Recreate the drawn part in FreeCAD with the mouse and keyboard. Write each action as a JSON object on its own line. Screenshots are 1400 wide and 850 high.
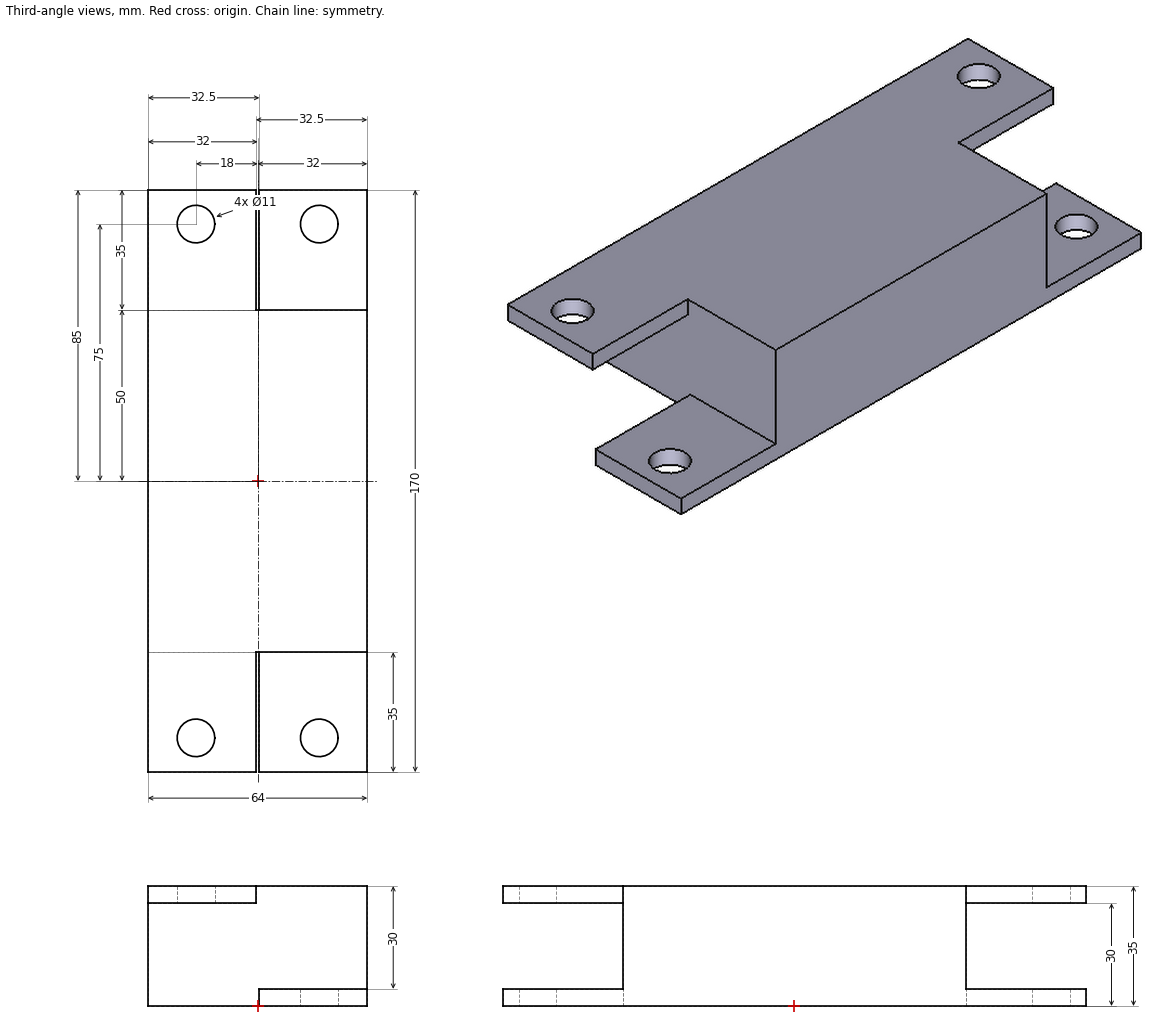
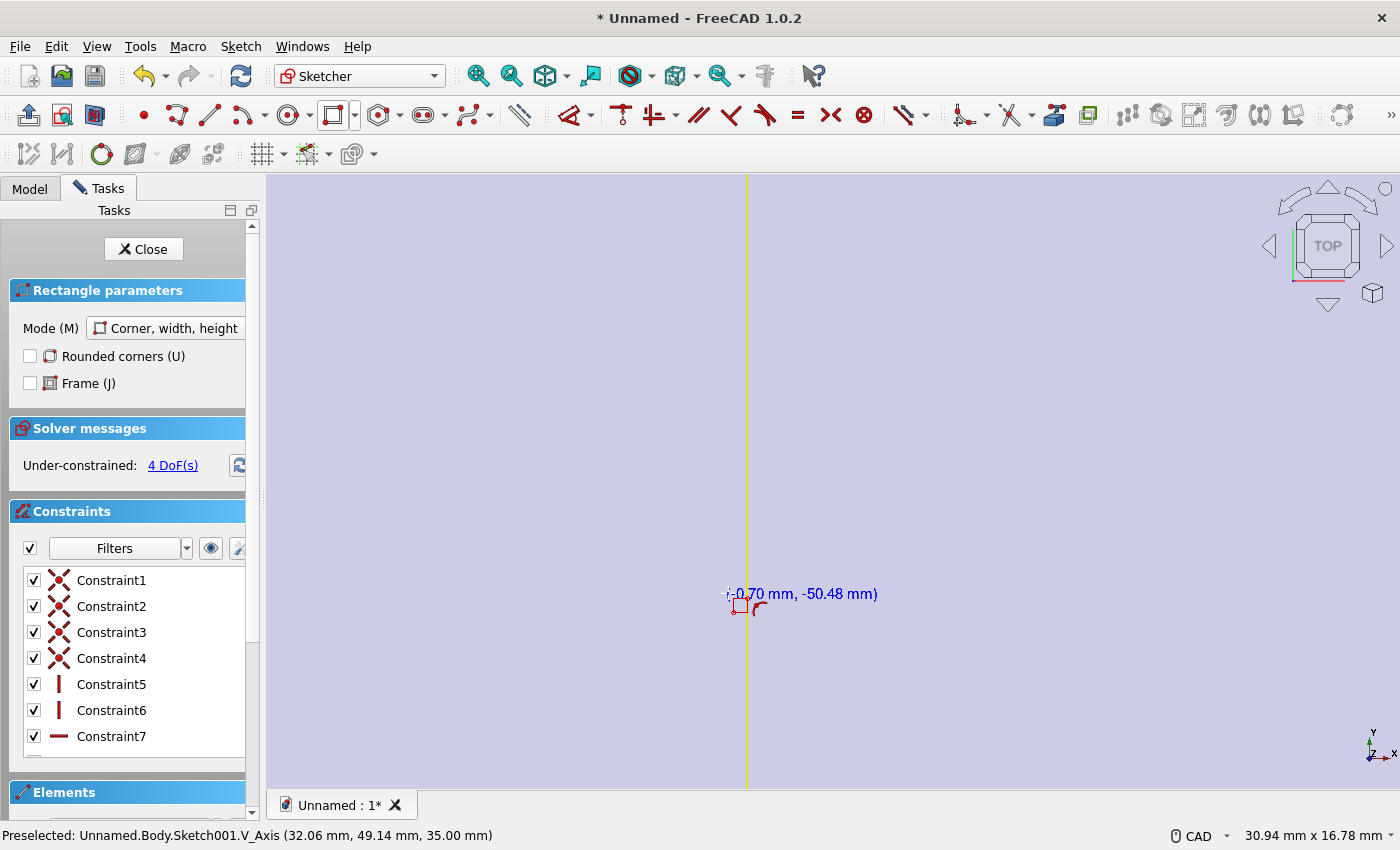
{"action": "left_click", "coordinate": [729, 581]}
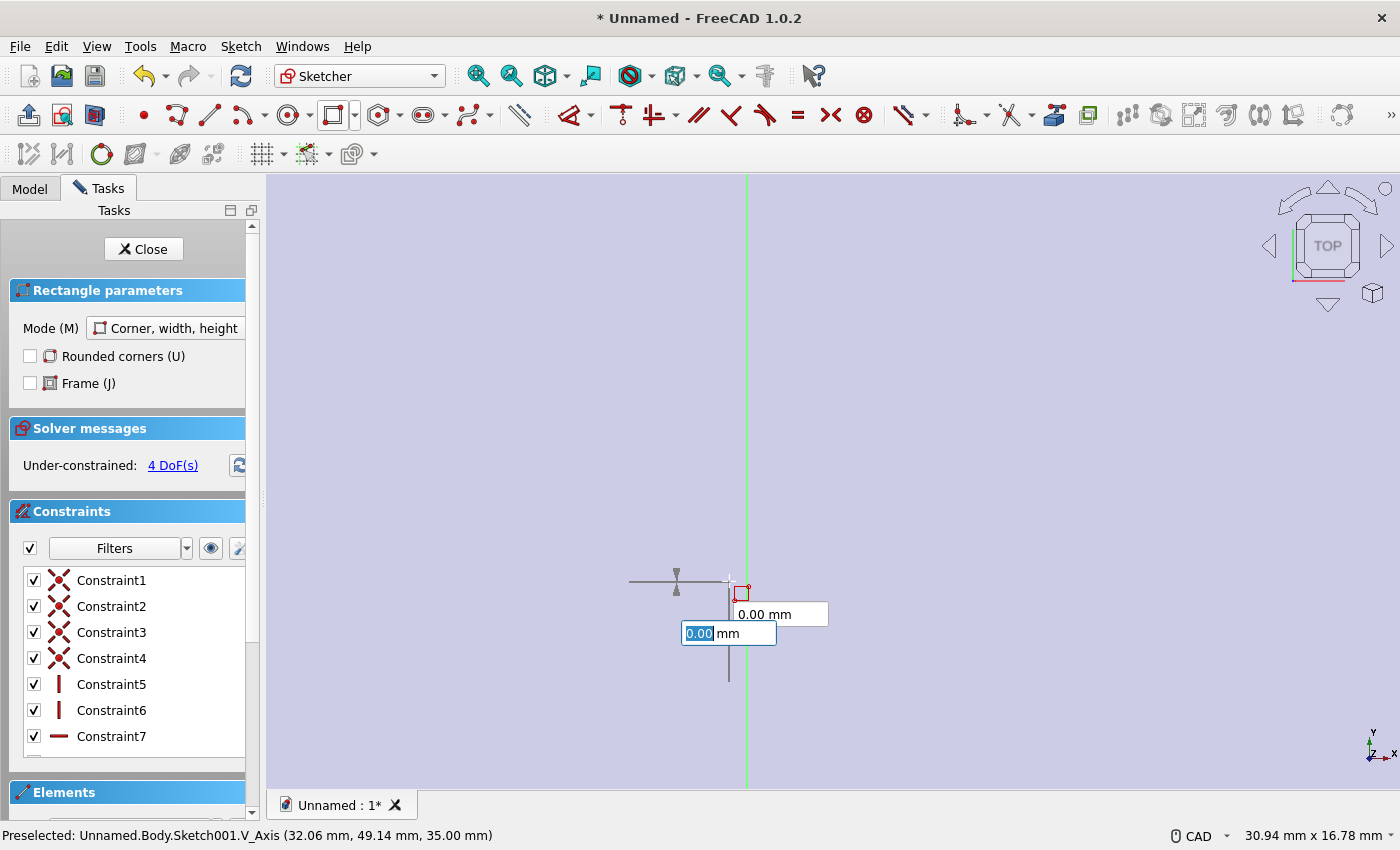
{"action": "scroll", "coordinate": [728, 594], "scroll_direction": "down", "scroll_amount": 14}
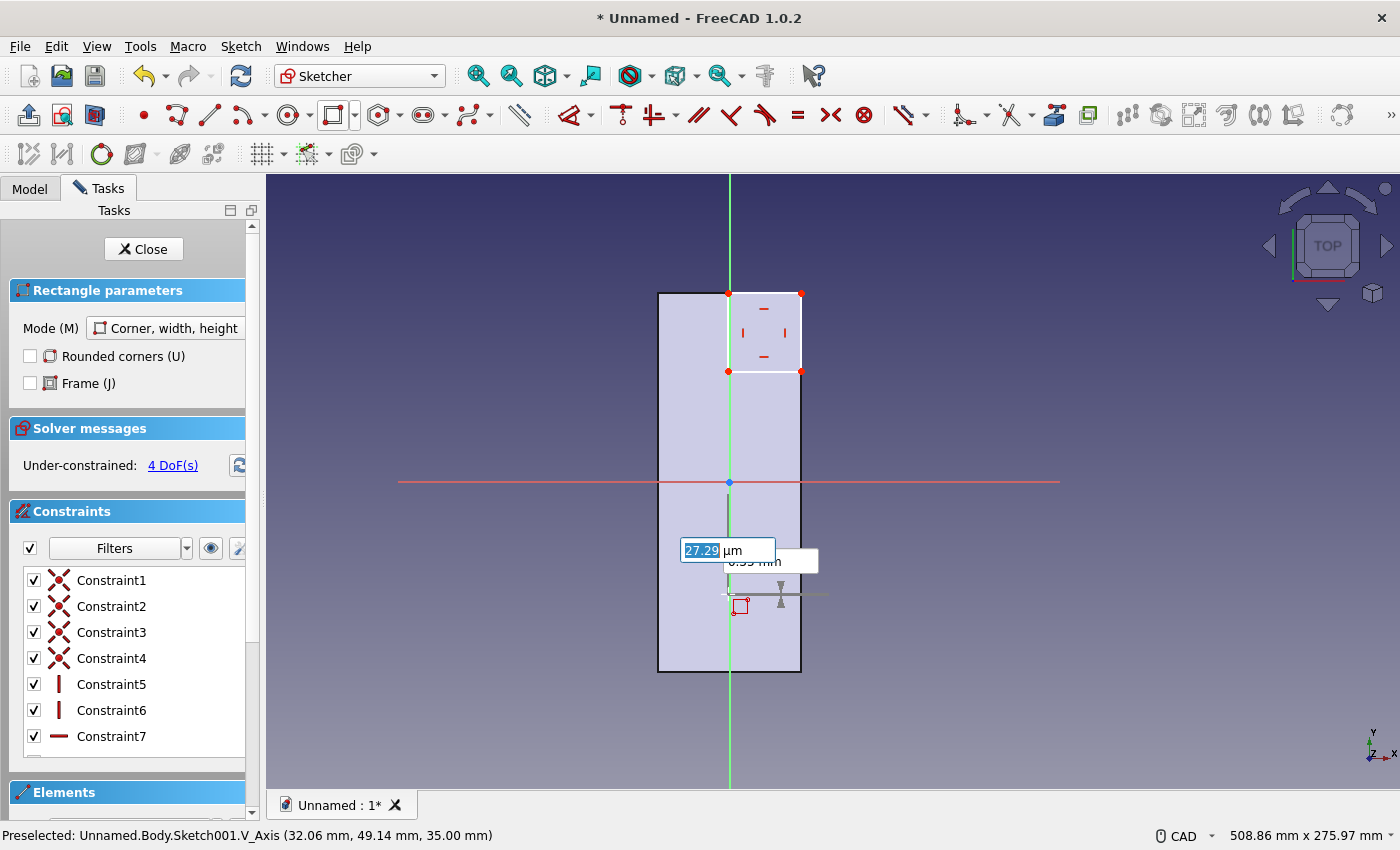
{"action": "left_click", "coordinate": [801, 672]}
{"action": "key", "text": "Escape"}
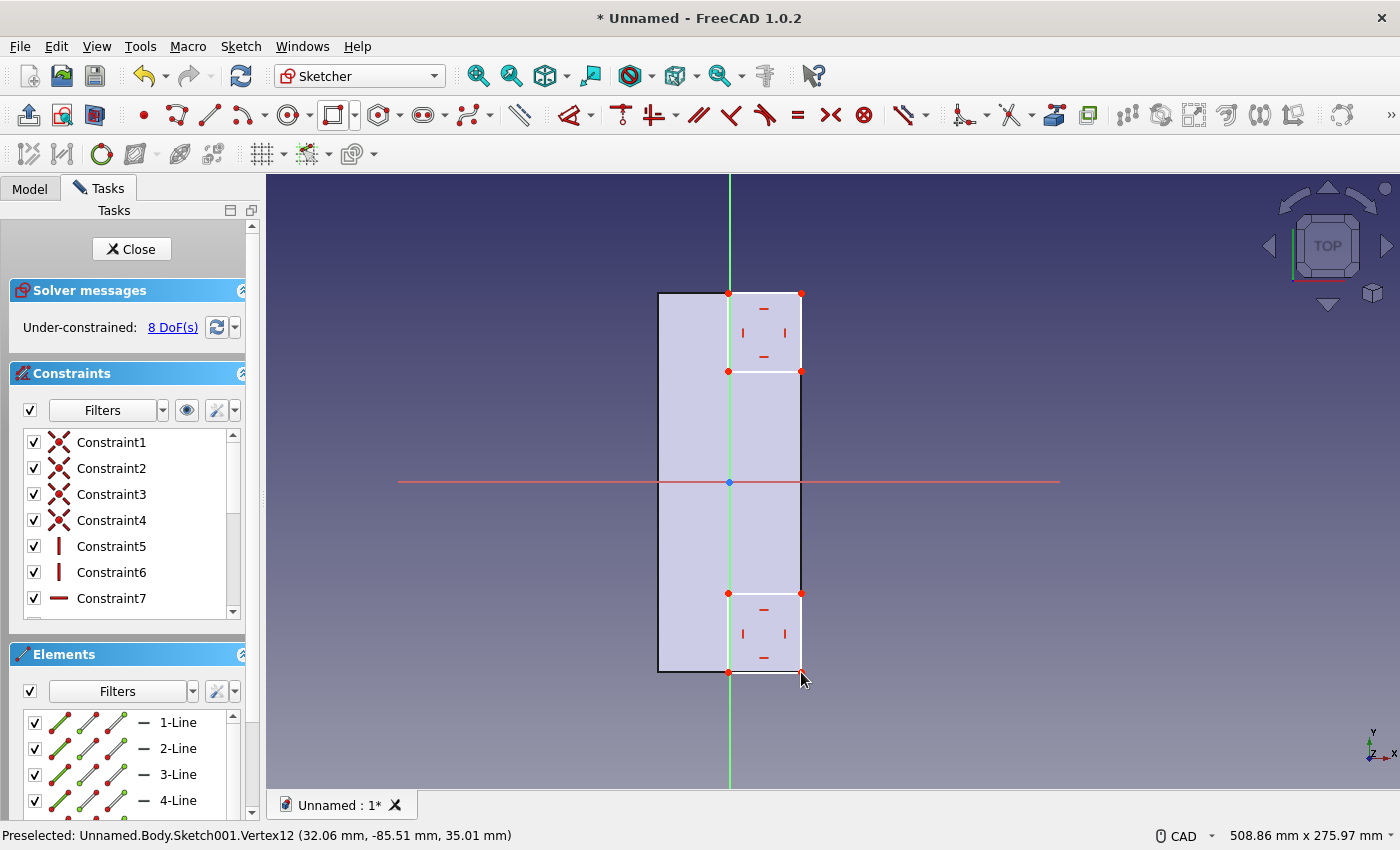
{"action": "left_click", "coordinate": [728, 372]}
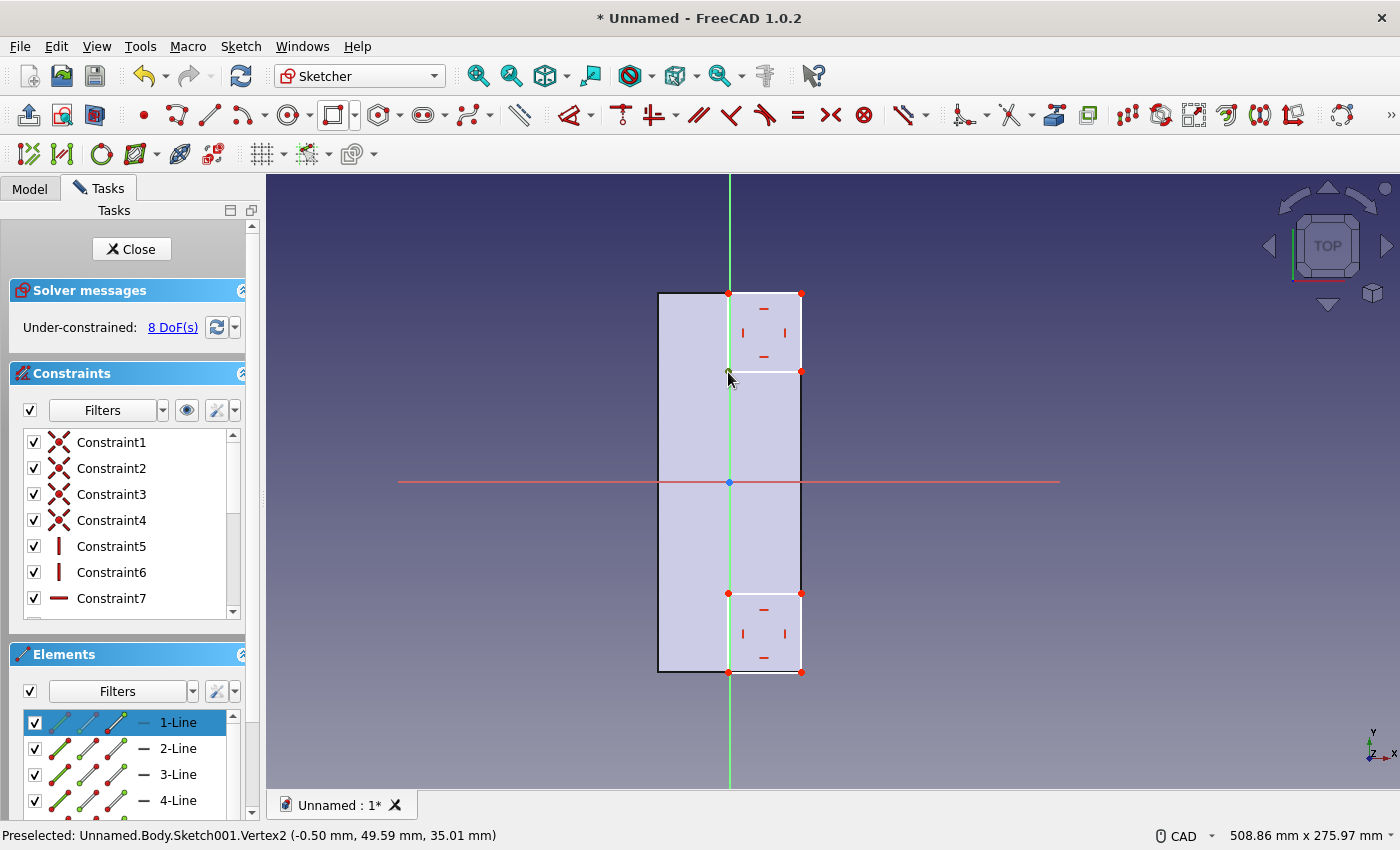
{"action": "left_click", "coordinate": [728, 594]}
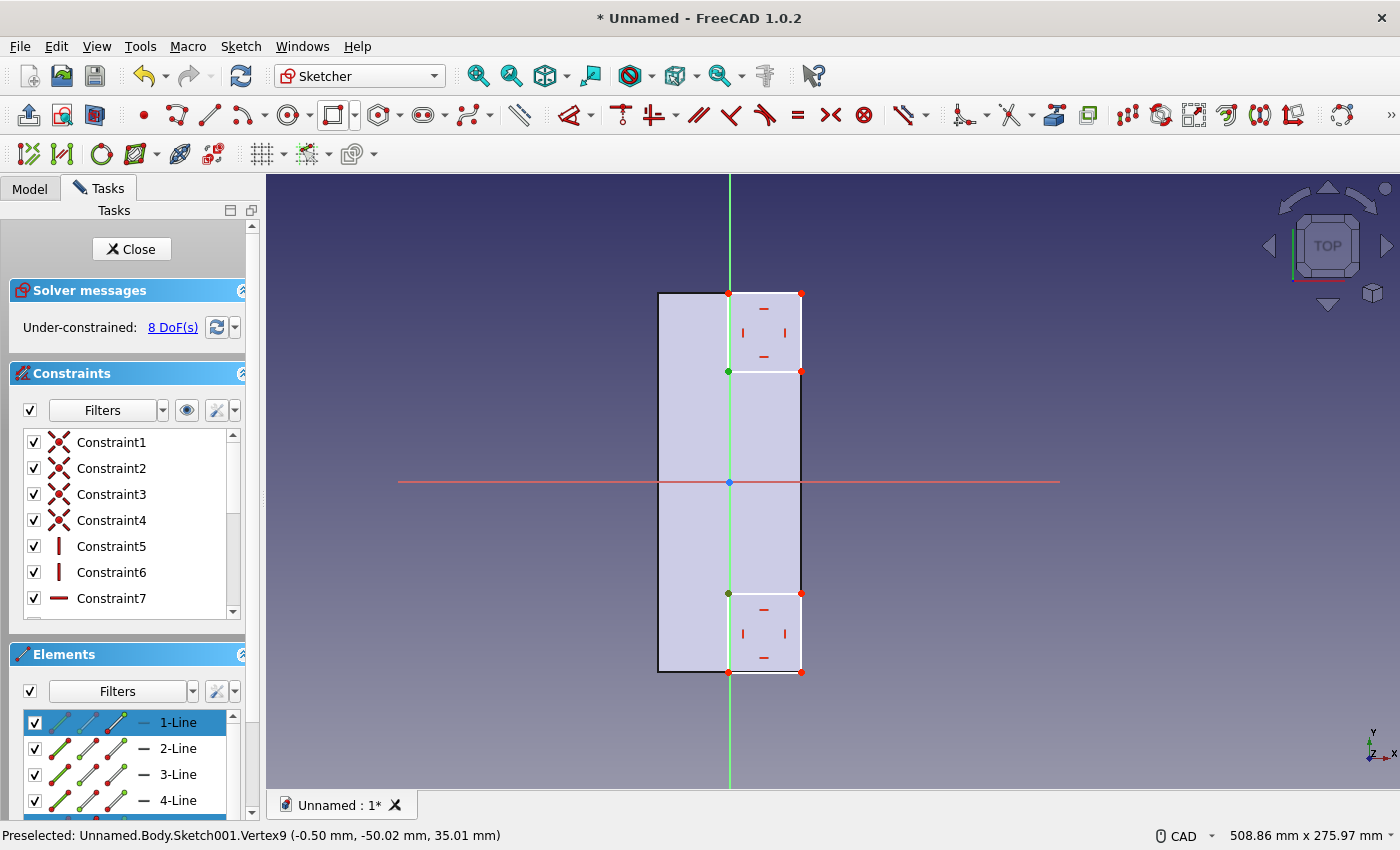
{"action": "left_click", "coordinate": [428, 482]}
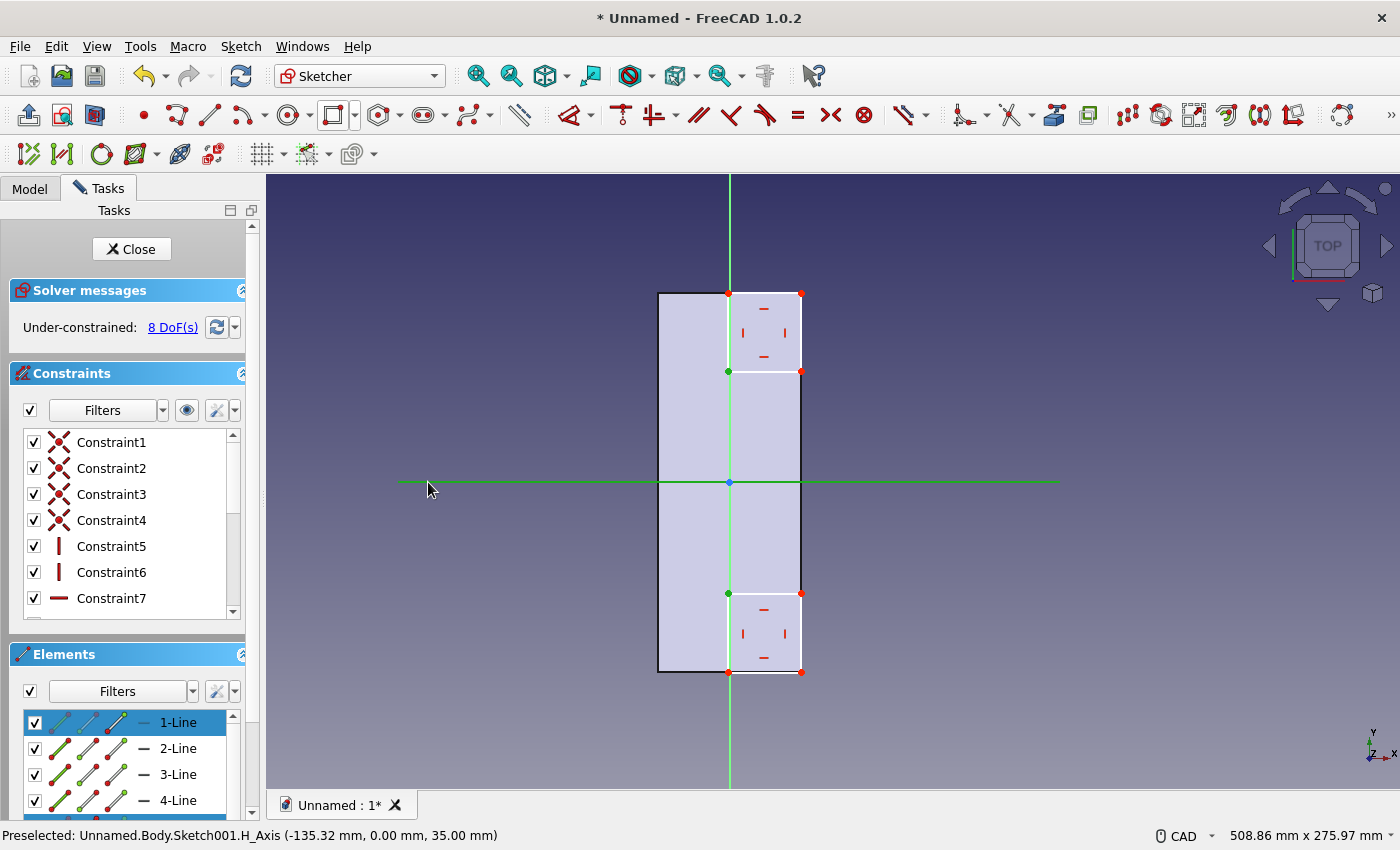
{"action": "left_click", "coordinate": [831, 116]}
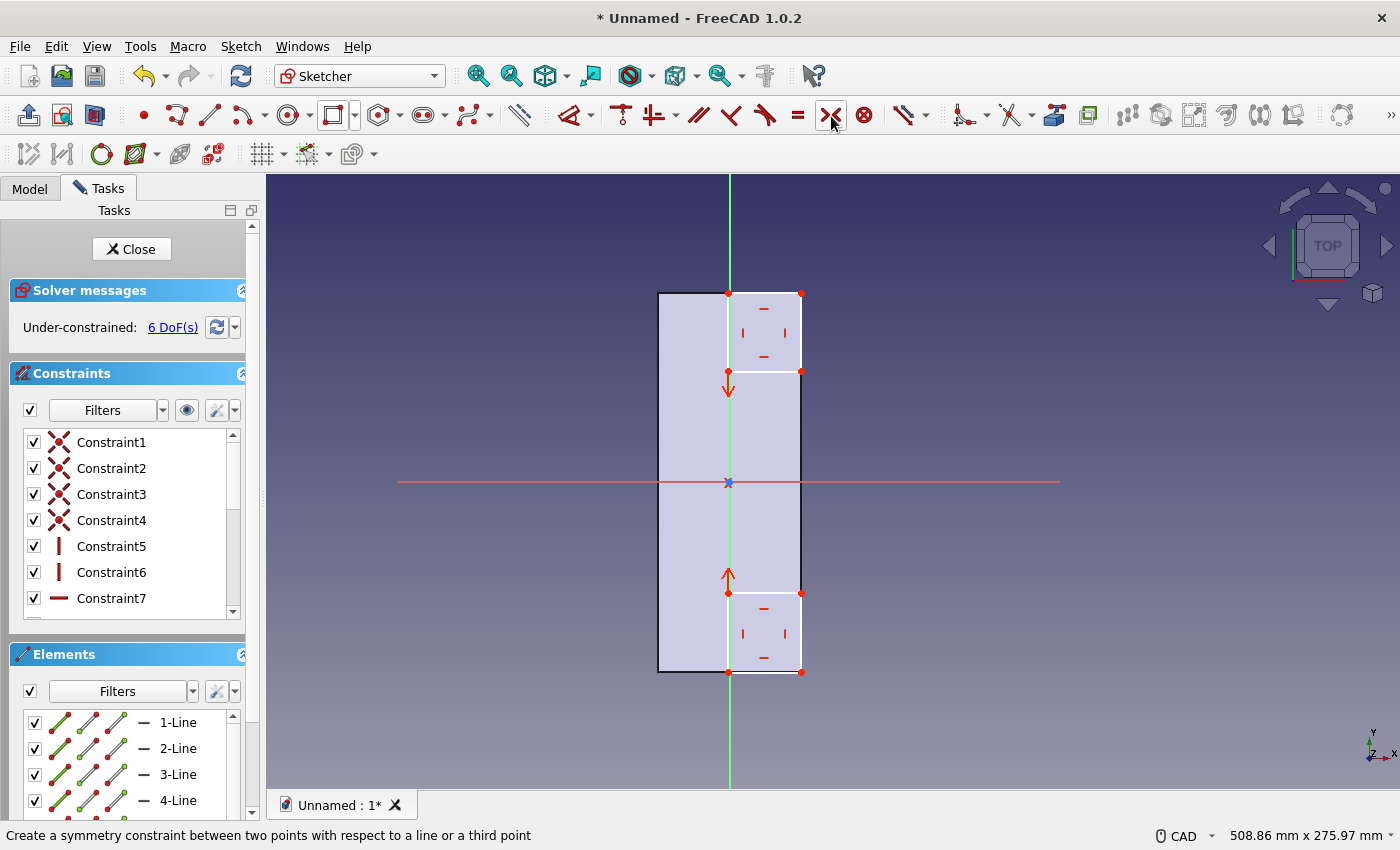
{"action": "left_click", "coordinate": [801, 293]}